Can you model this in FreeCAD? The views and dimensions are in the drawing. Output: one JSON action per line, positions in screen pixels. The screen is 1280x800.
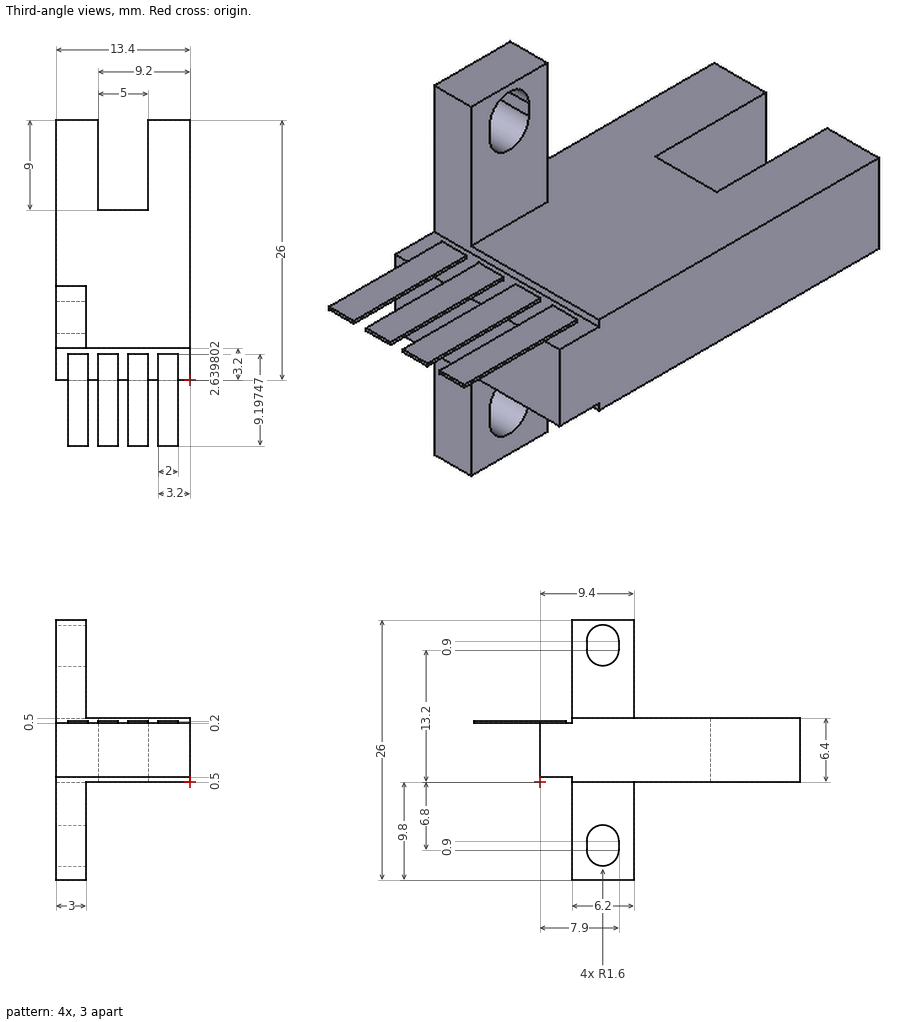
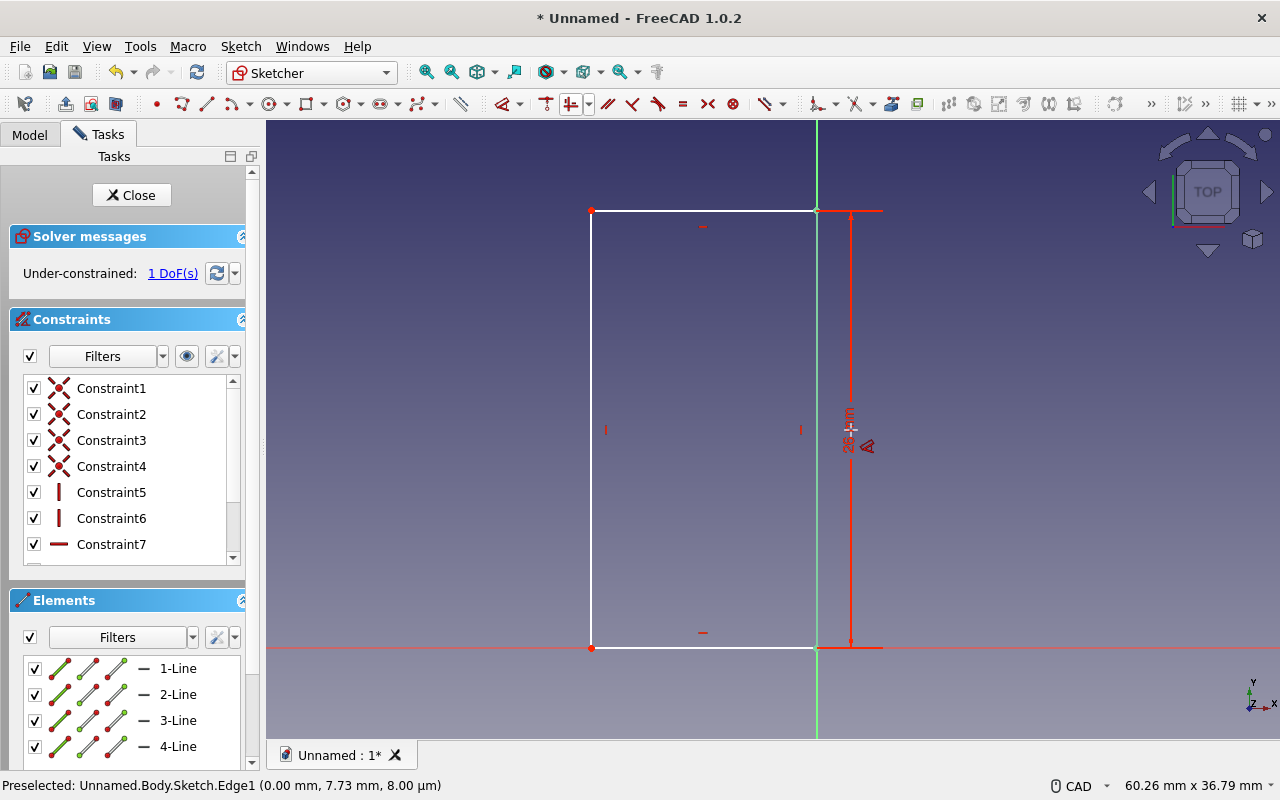
{"action": "left_click", "coordinate": [749, 211]}
{"action": "left_click", "coordinate": [704, 177]}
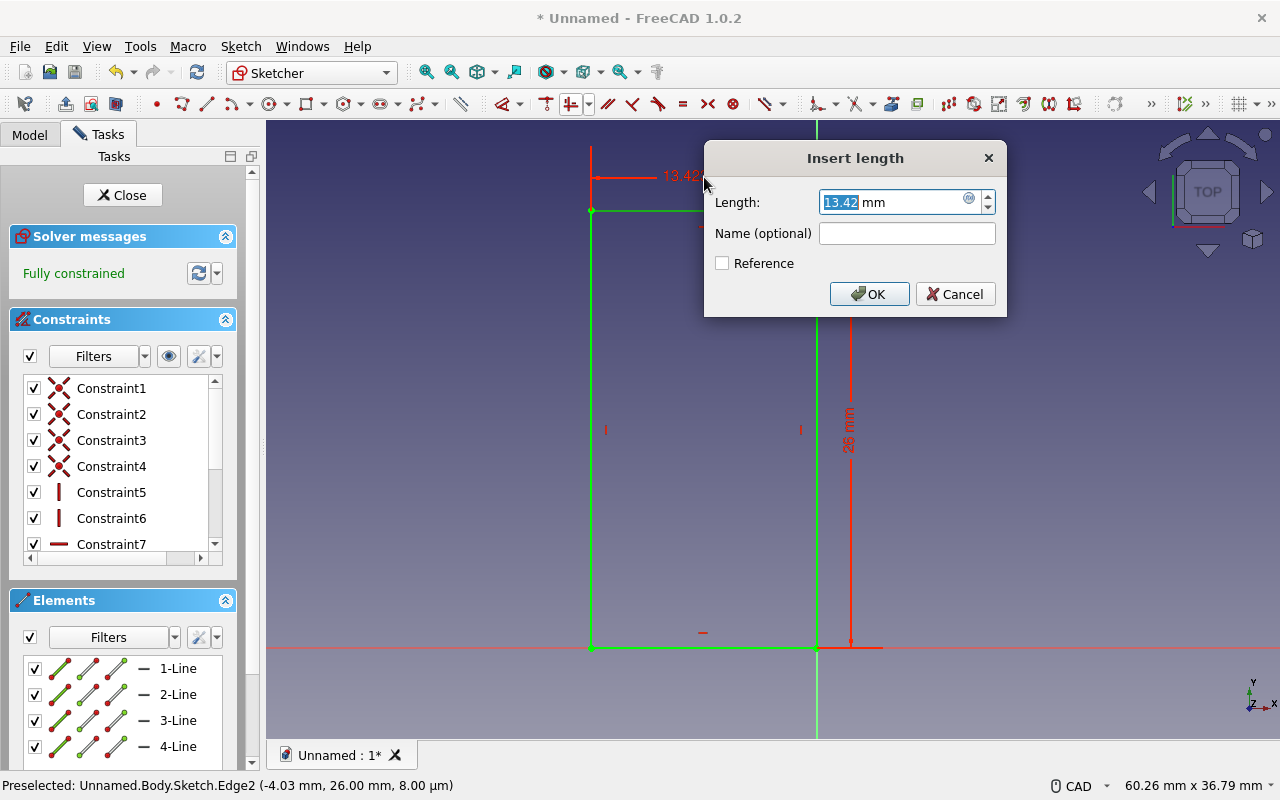
{"action": "type", "text": "13.4"}
{"action": "key", "text": "Return"}
{"action": "key", "text": "Escape"}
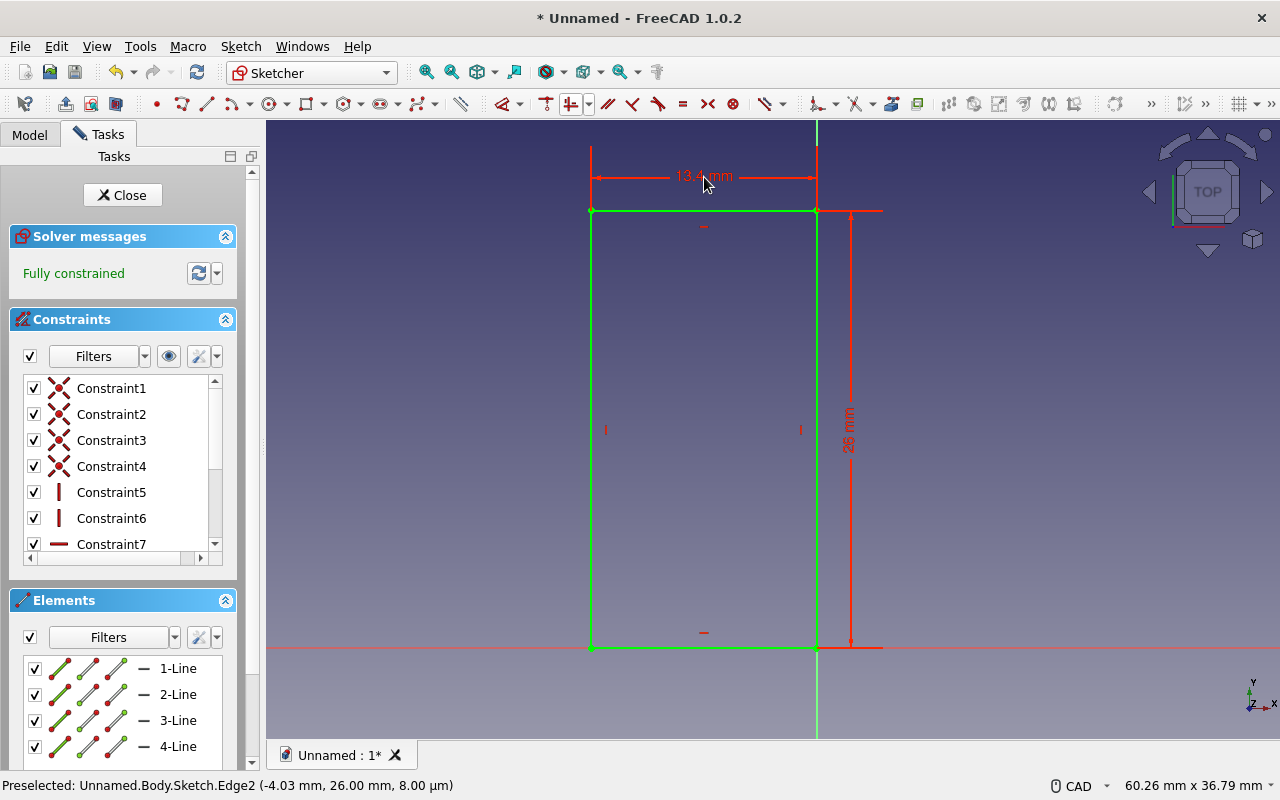
{"action": "left_click", "coordinate": [123, 195]}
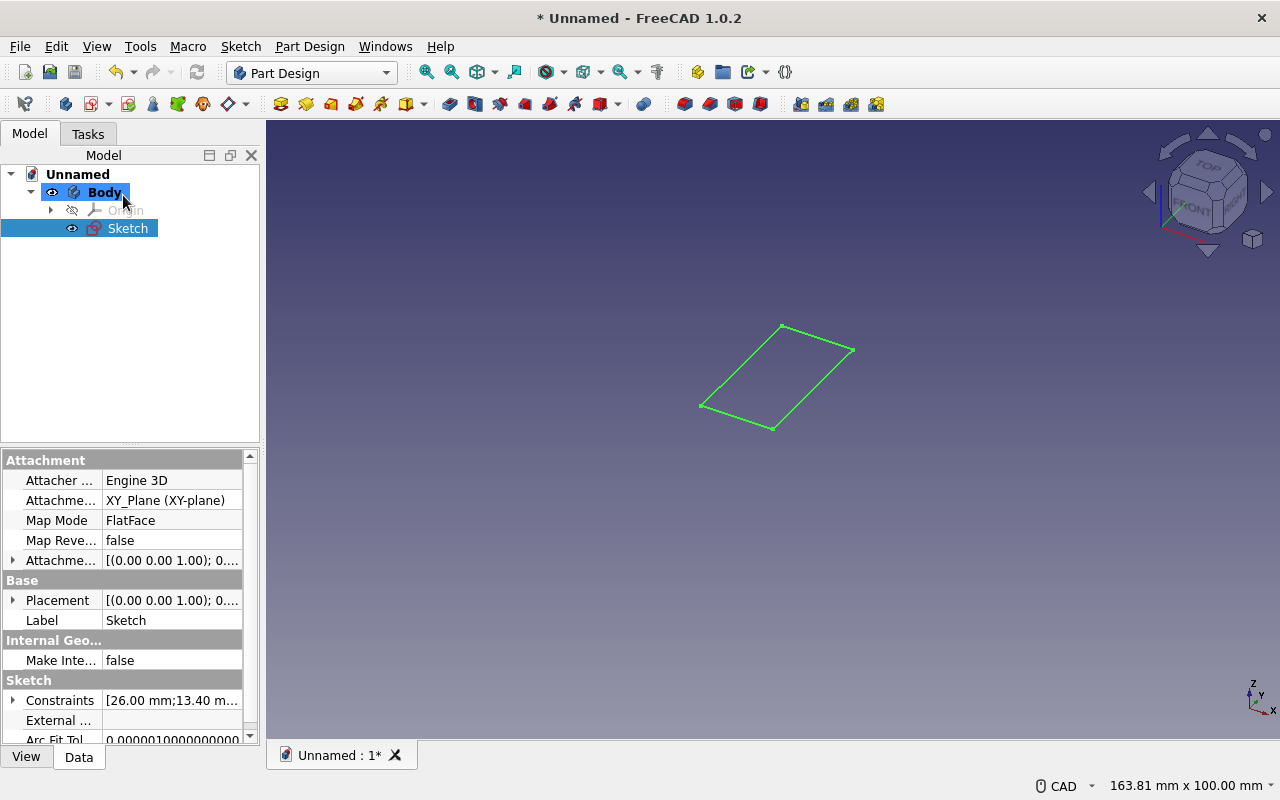
{"action": "left_click", "coordinate": [281, 104]}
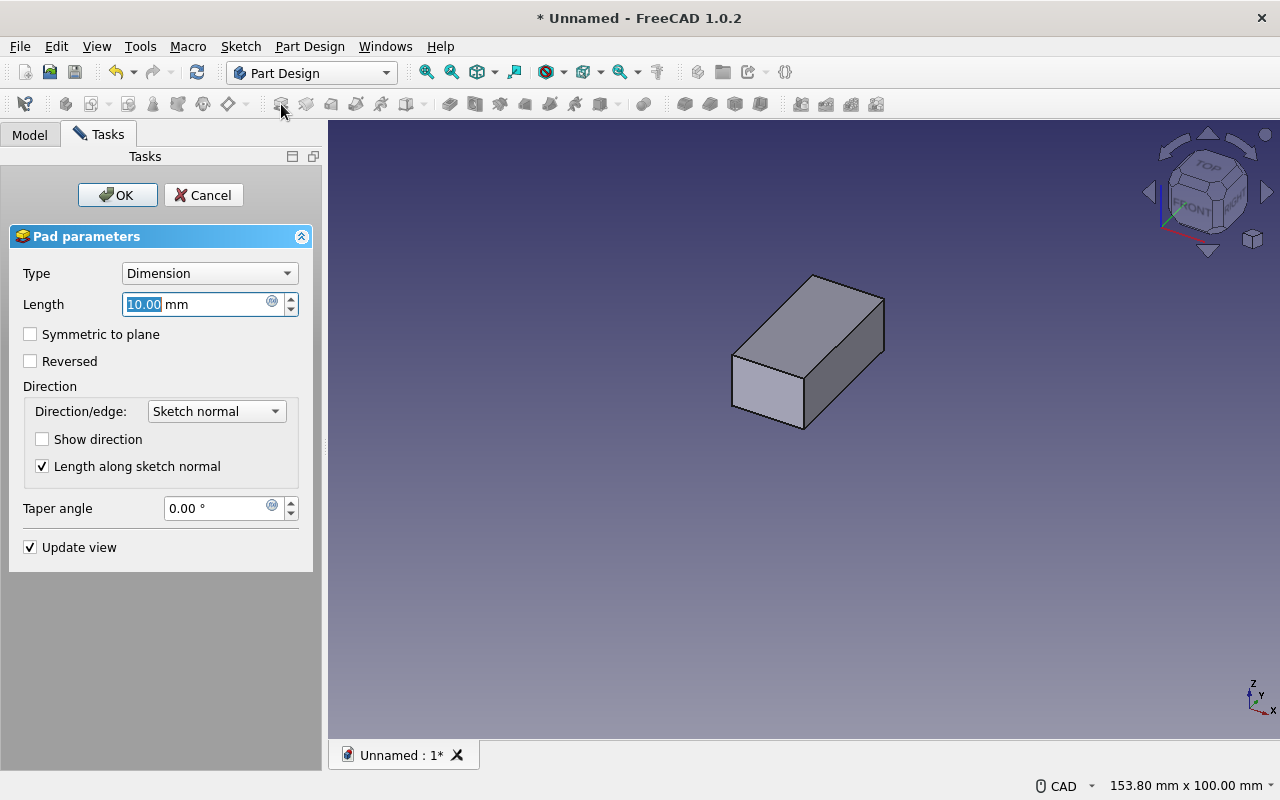
{"action": "type", "text": "6.4"}
{"action": "key", "text": "Tab"}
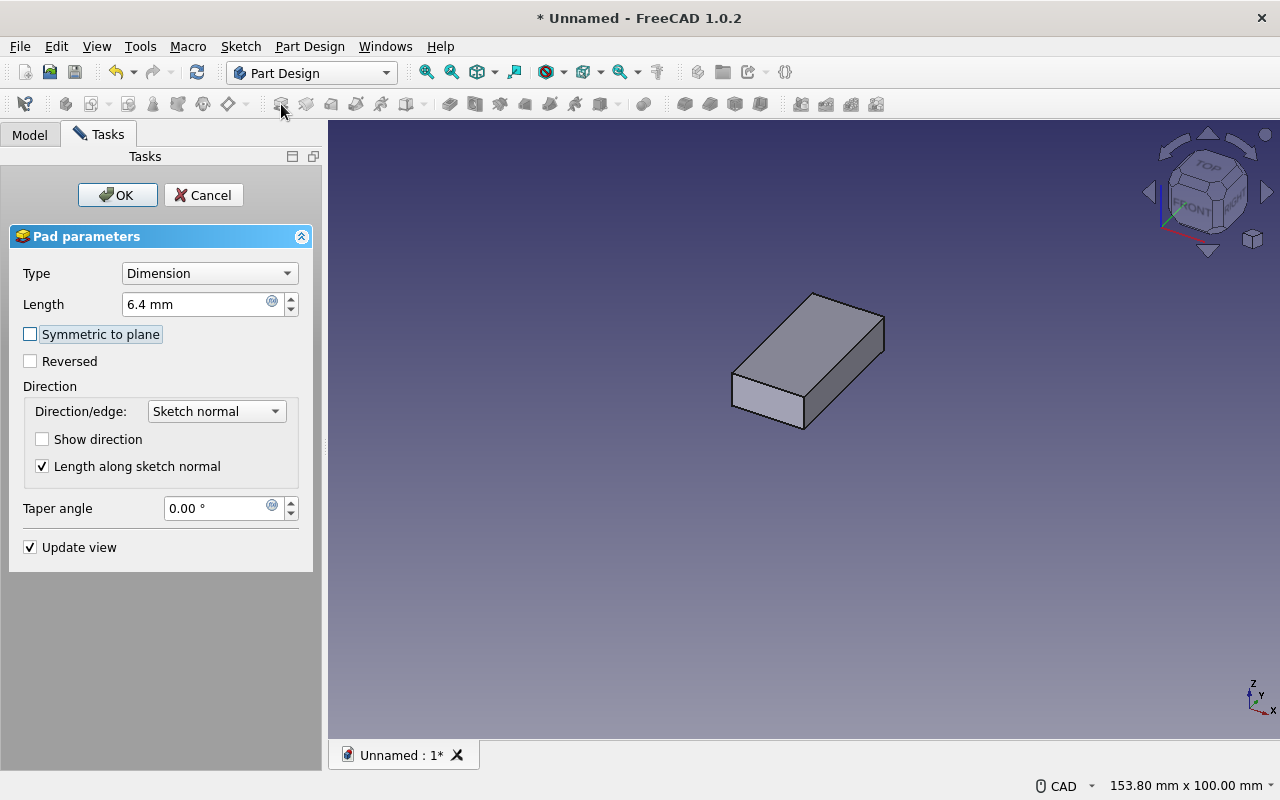
{"action": "left_click", "coordinate": [118, 195]}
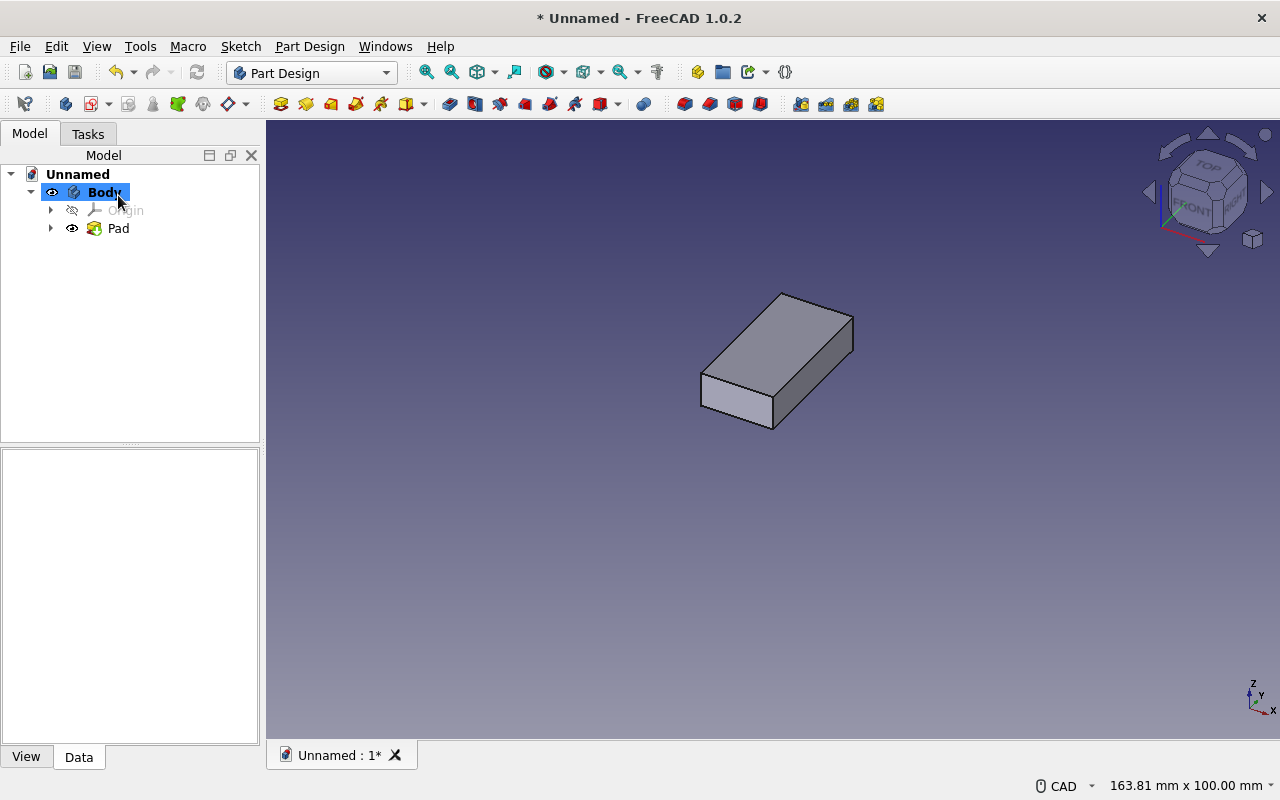
{"action": "left_click", "coordinate": [427, 72]}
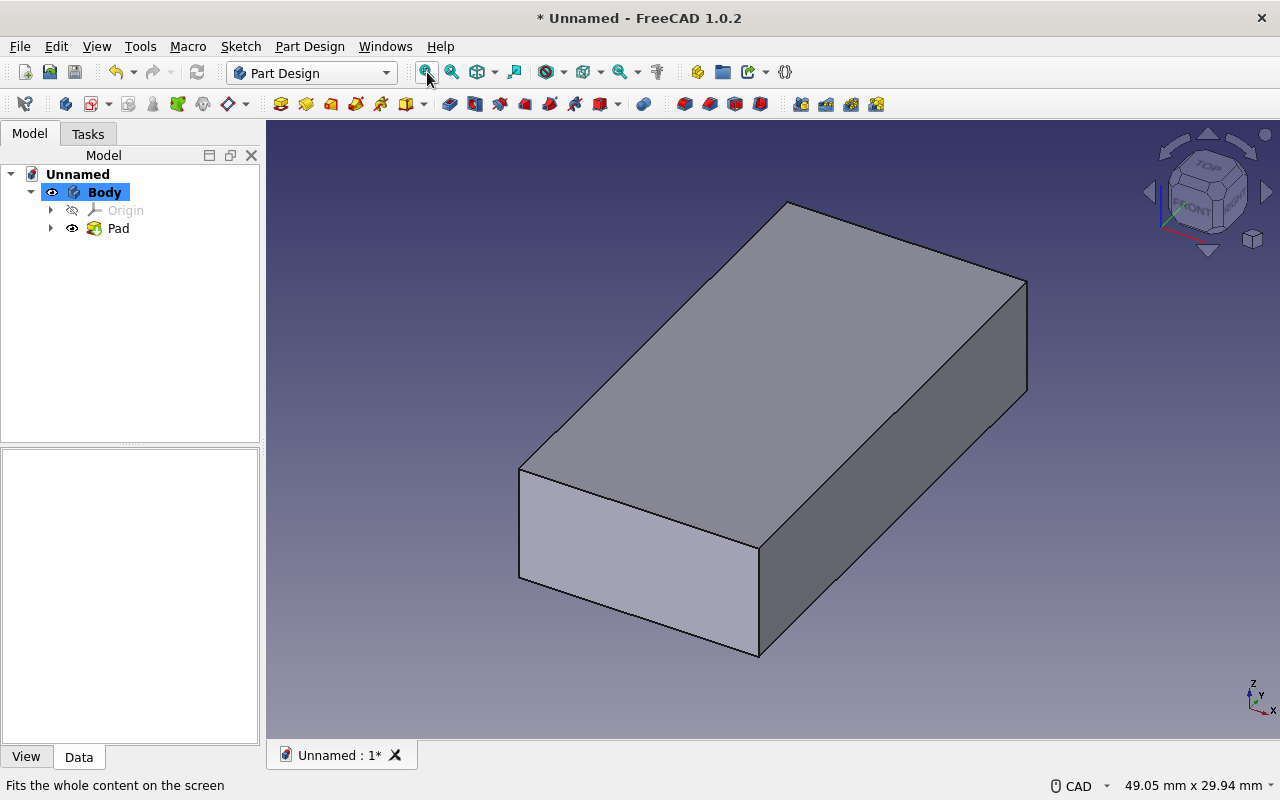
{"action": "left_click", "coordinate": [811, 336]}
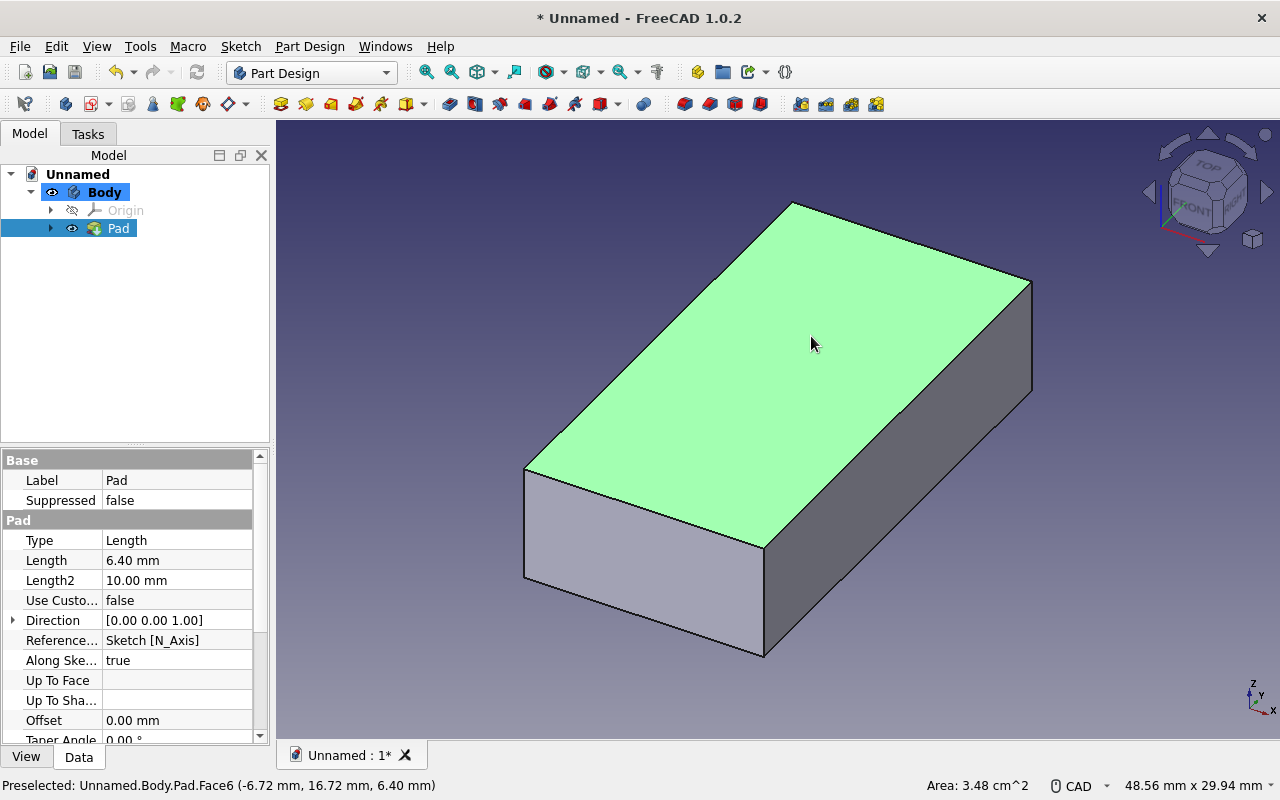
{"action": "left_click", "coordinate": [90, 104]}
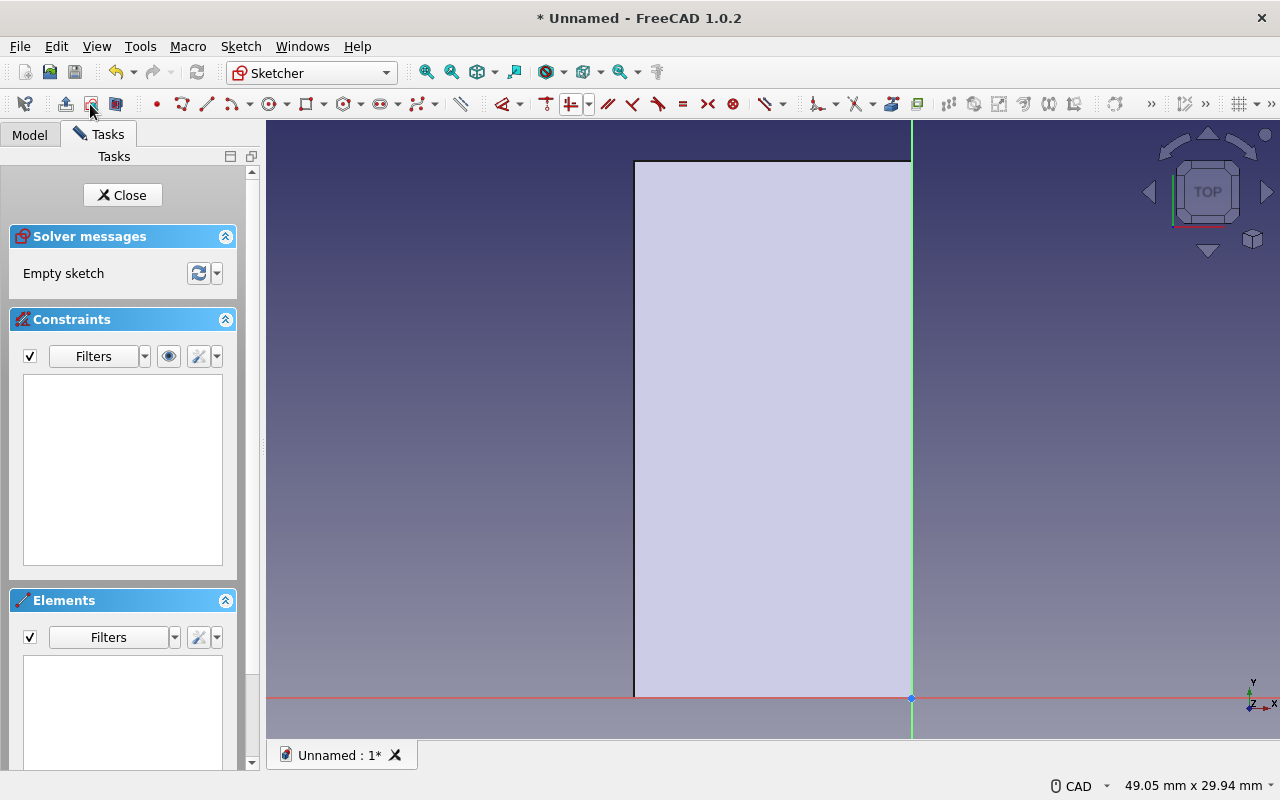
{"action": "scroll", "coordinate": [829, 148], "scroll_direction": "up", "scroll_amount": 4}